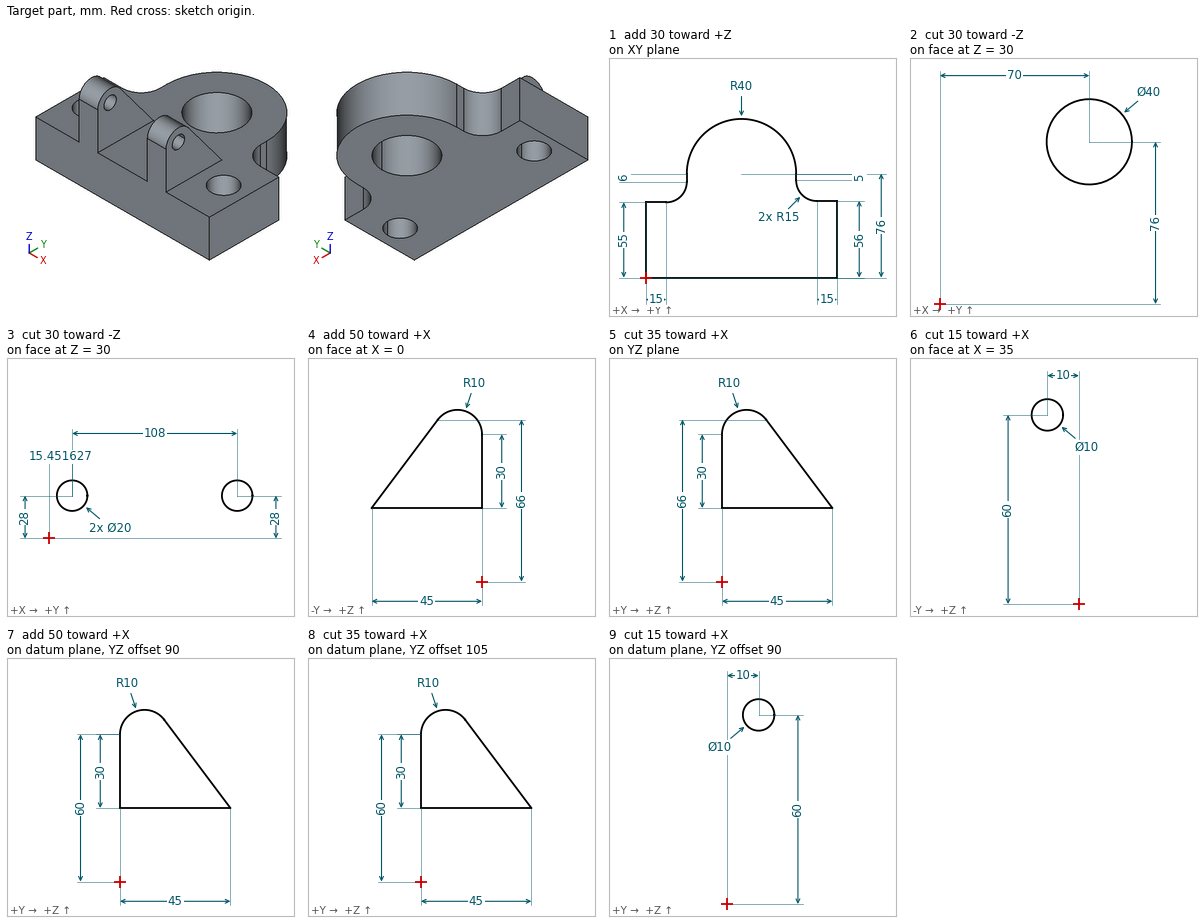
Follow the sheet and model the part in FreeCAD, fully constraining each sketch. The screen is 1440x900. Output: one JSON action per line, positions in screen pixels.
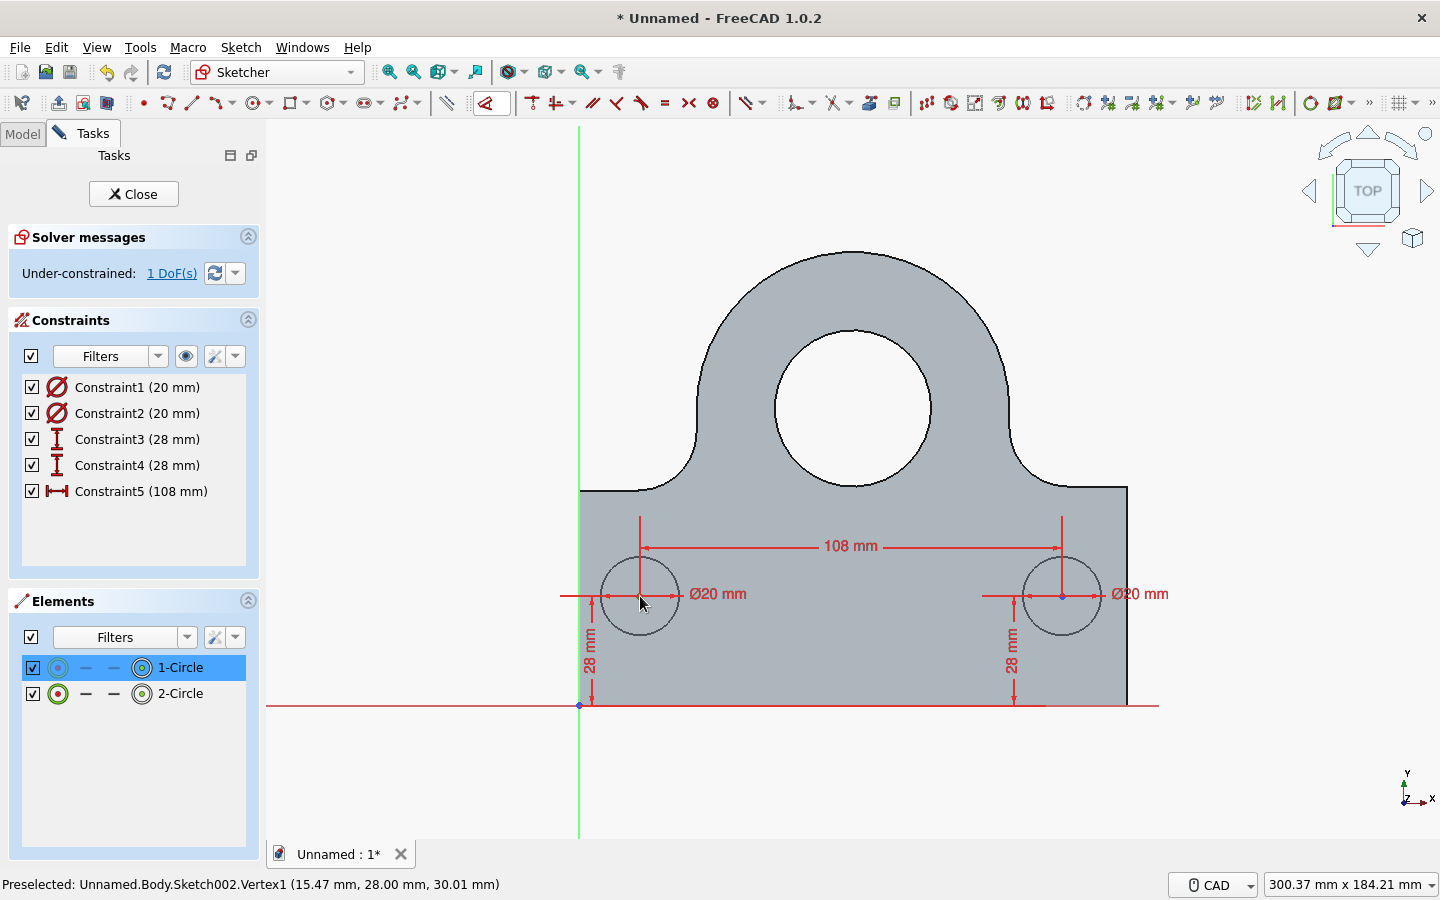
{"action": "key", "text": "l"}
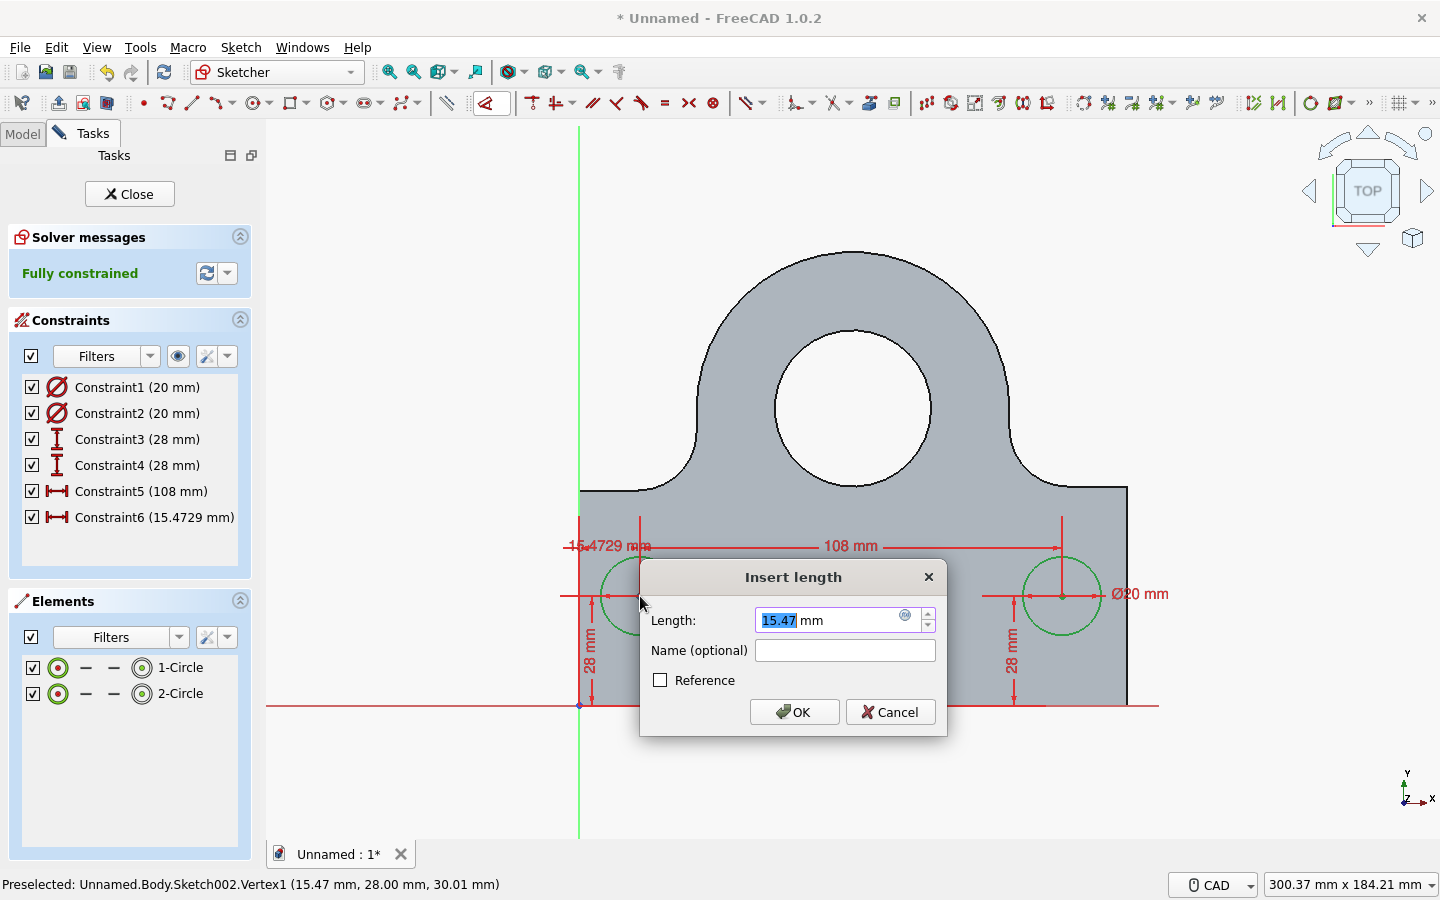
{"action": "type", "text": "15.451627"}
{"action": "key", "text": "Return"}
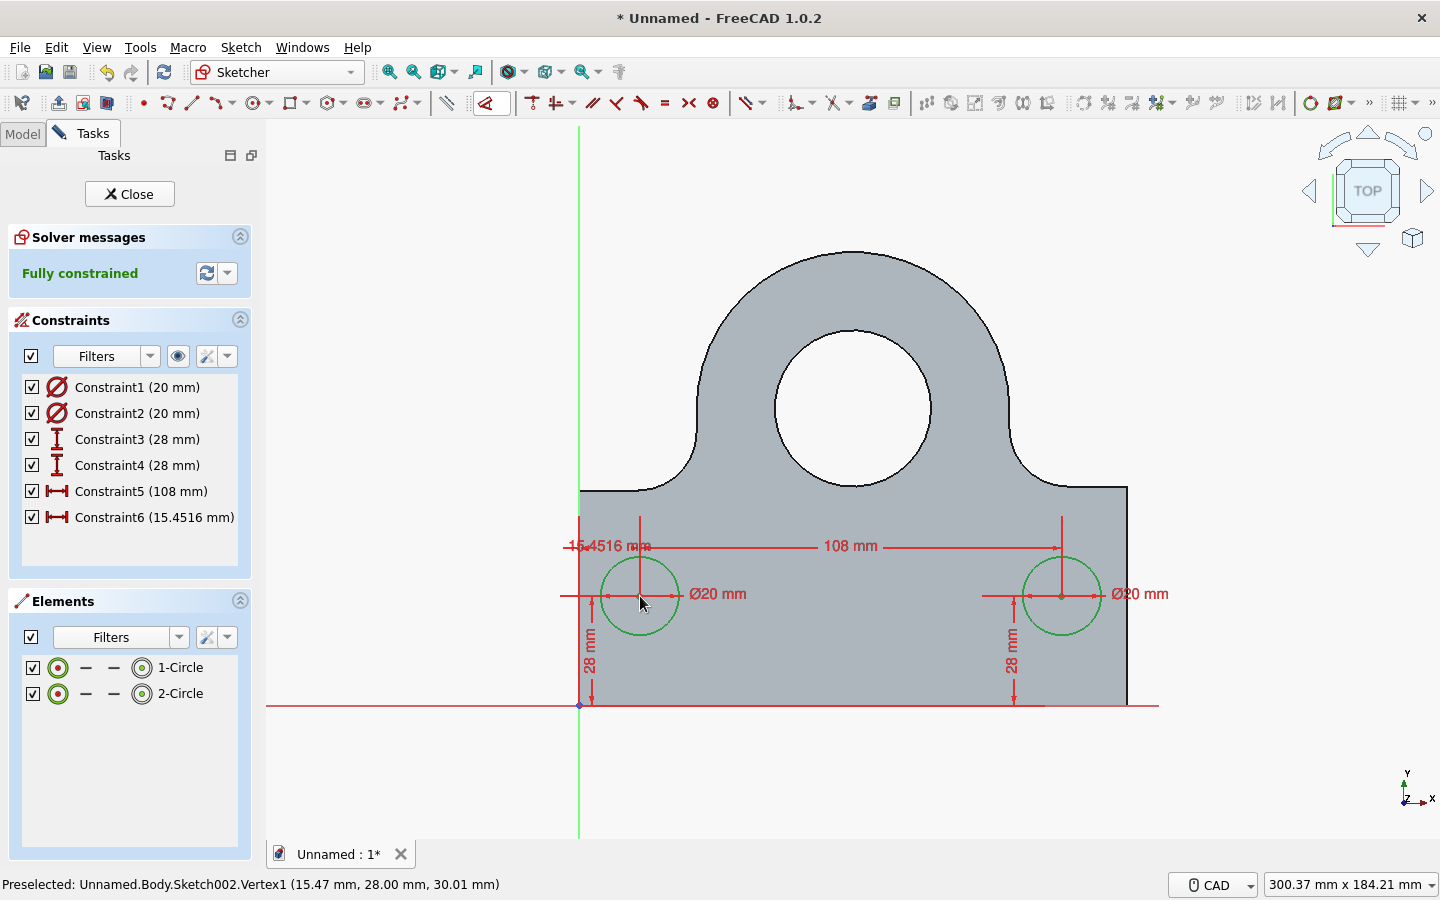
{"action": "left_click", "coordinate": [130, 194]}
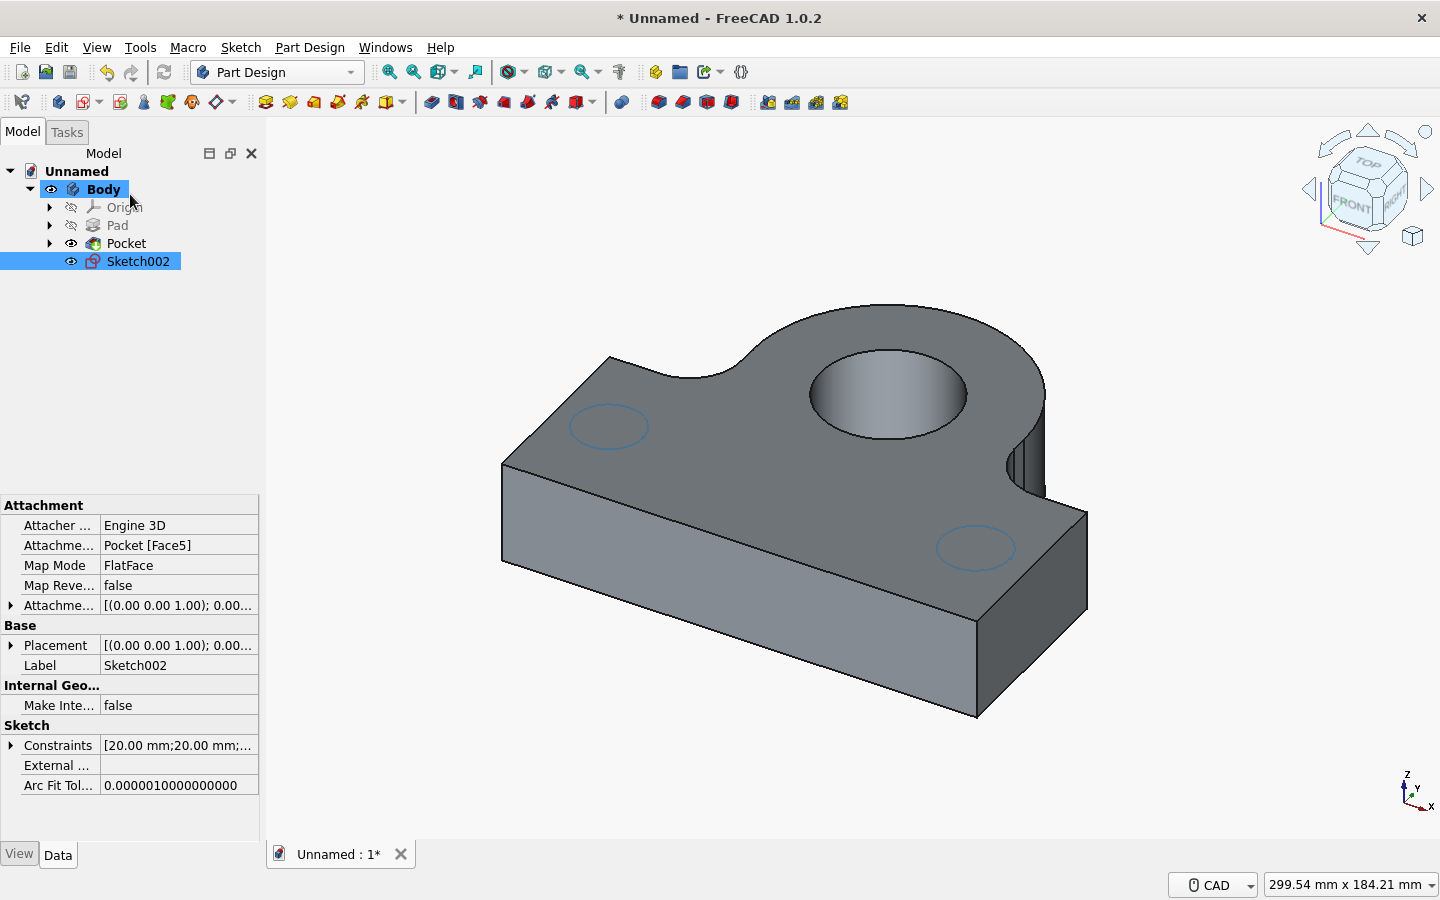
{"action": "left_click", "coordinate": [432, 102]}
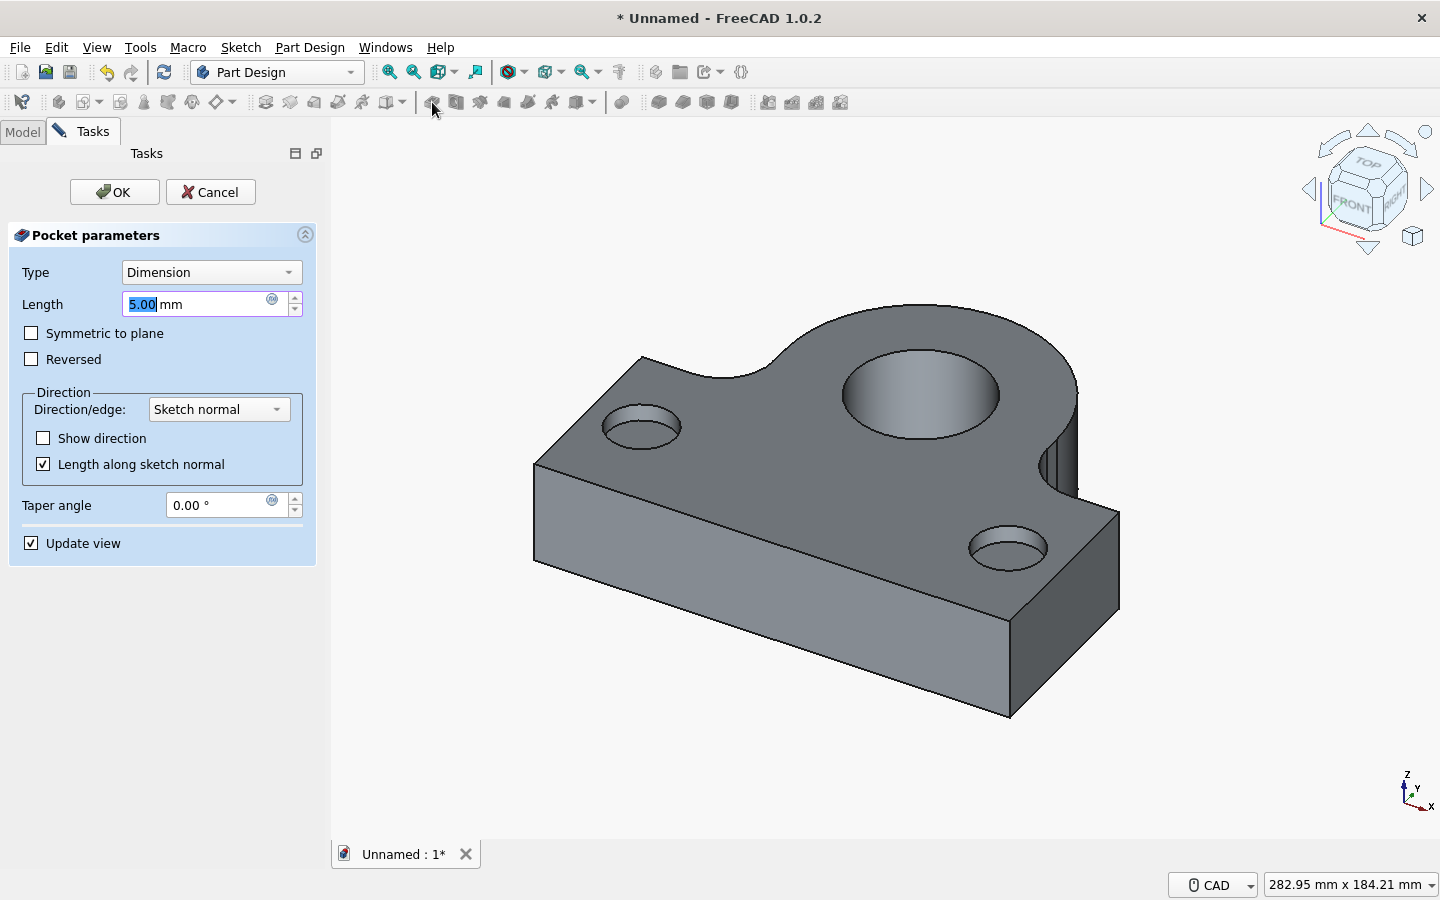
{"action": "type", "text": "30"}
{"action": "key", "text": "Tab"}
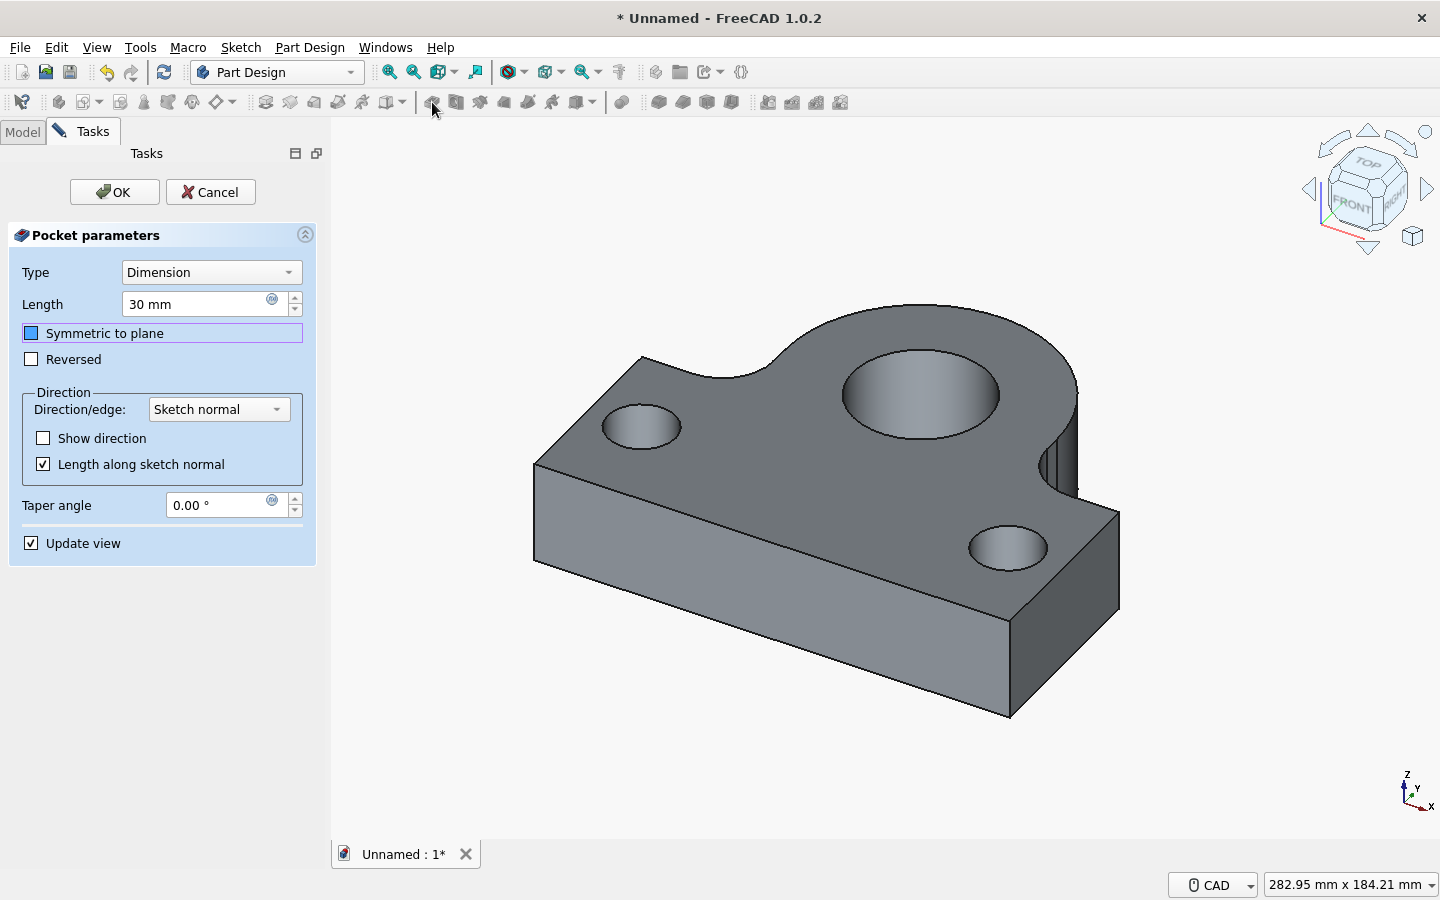
{"action": "left_click", "coordinate": [115, 192]}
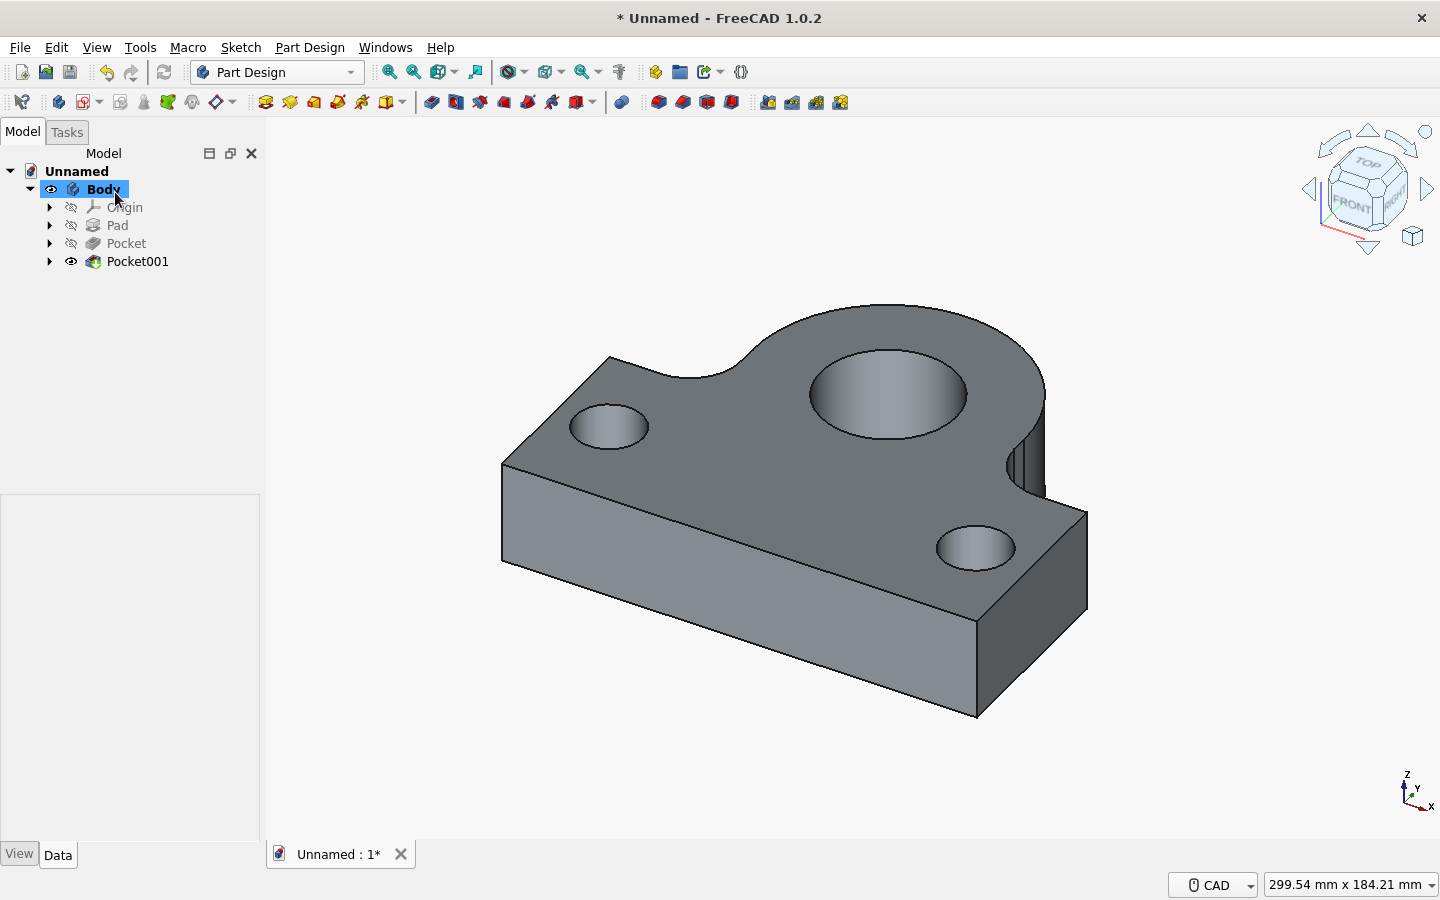
{"action": "key", "text": "6"}